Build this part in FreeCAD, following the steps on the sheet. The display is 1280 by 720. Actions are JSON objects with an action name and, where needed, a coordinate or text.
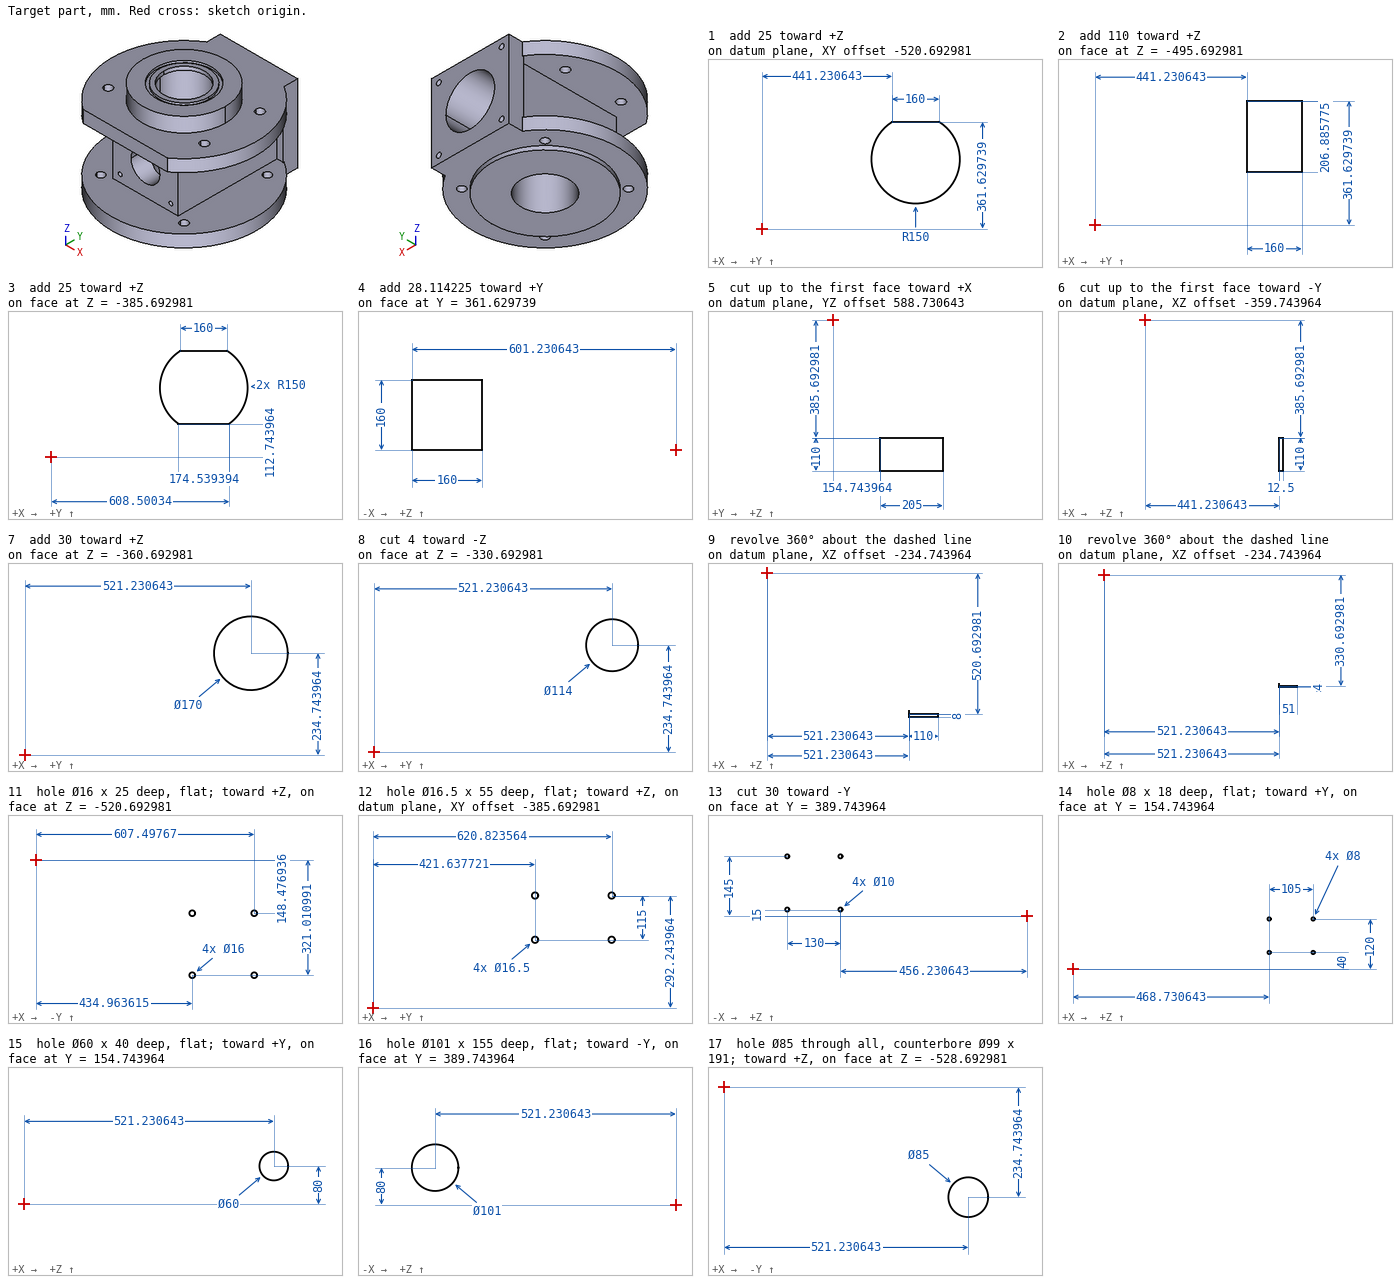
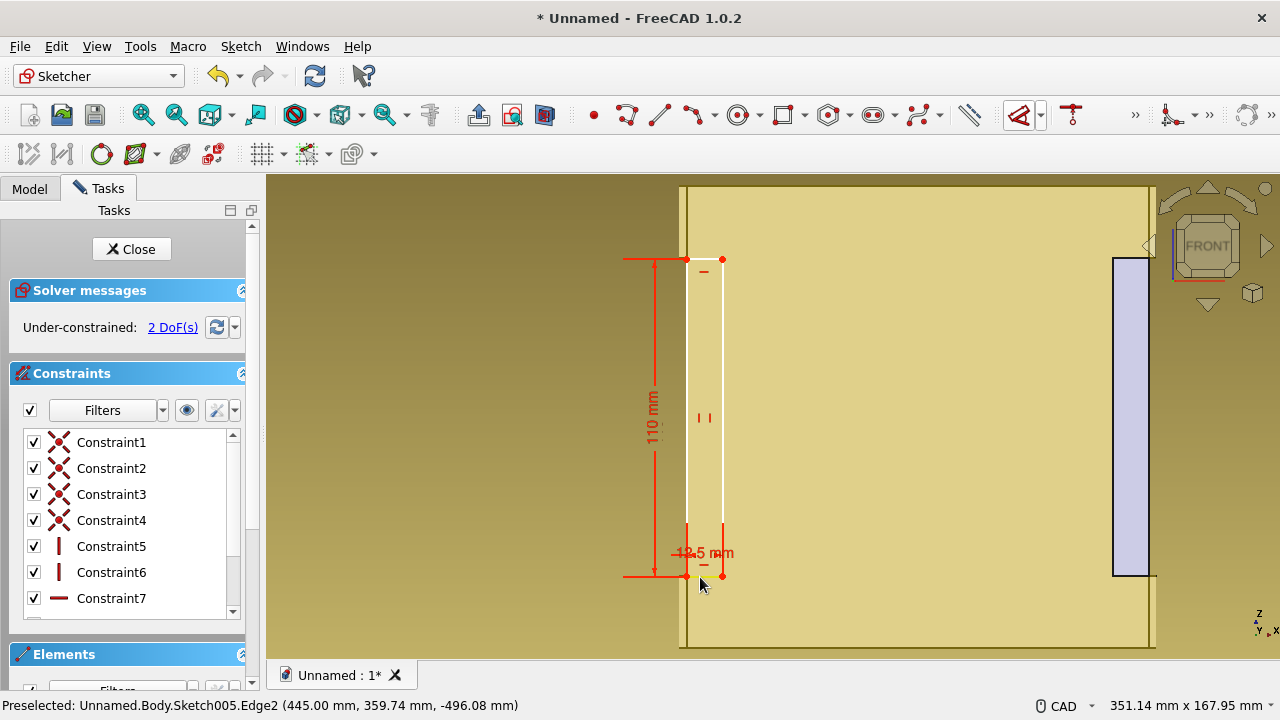
{"action": "left_click", "coordinate": [687, 259]}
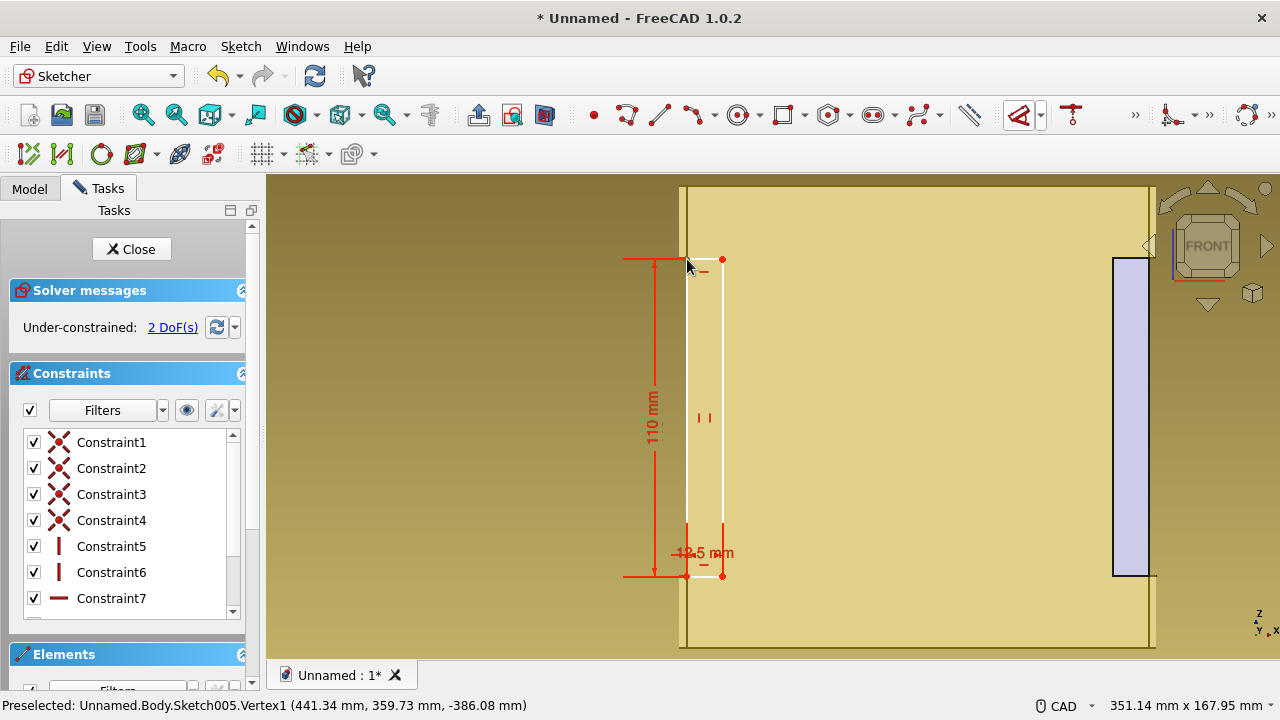
{"action": "left_click", "coordinate": [1040, 116]}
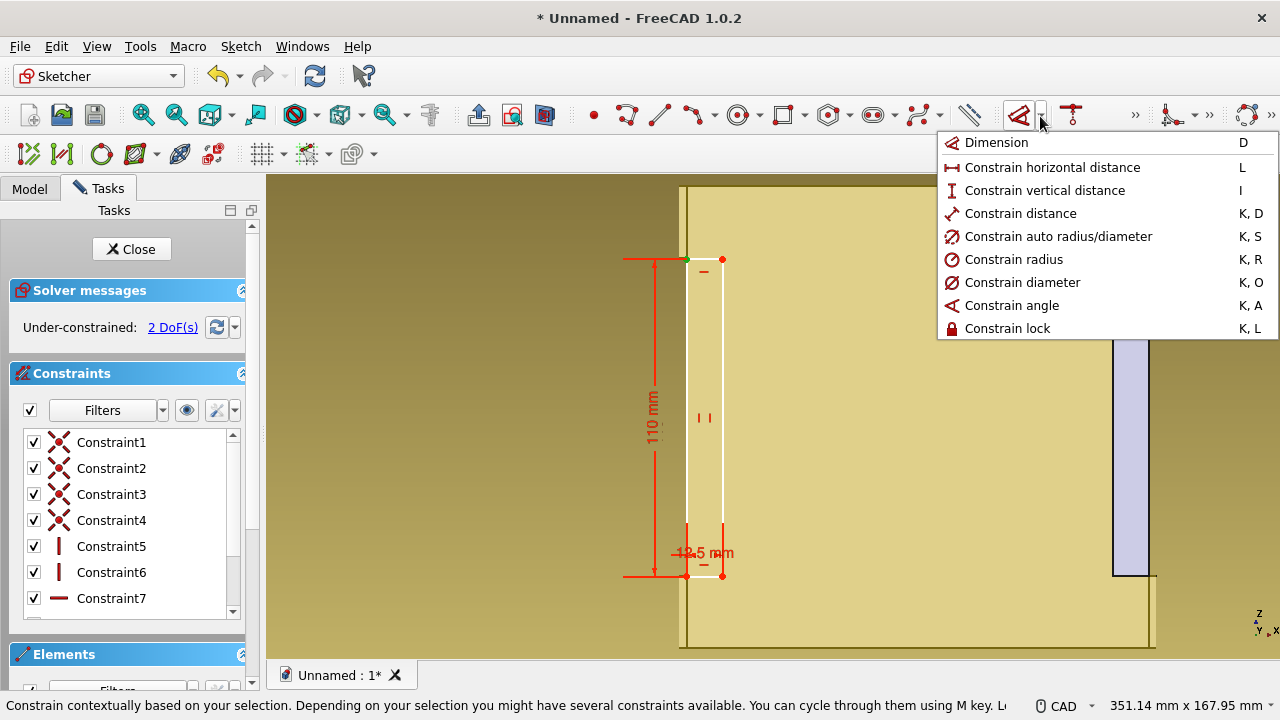
{"action": "left_click", "coordinate": [1108, 168]}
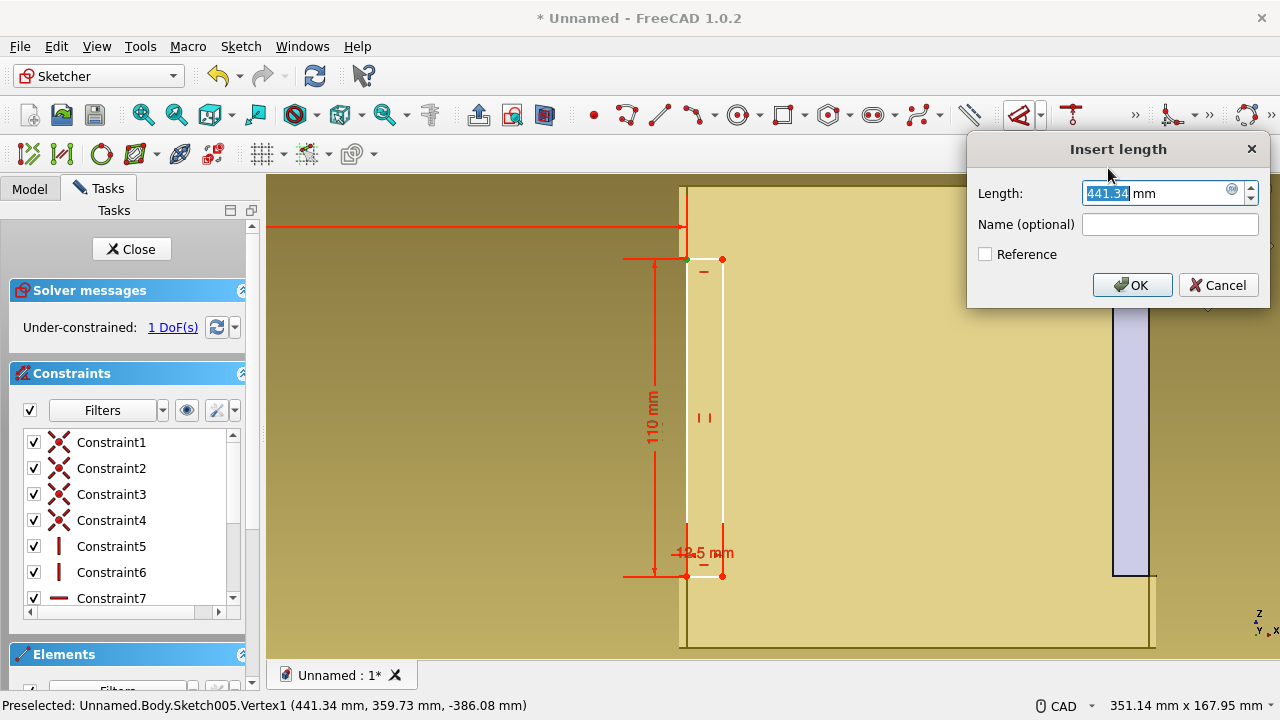
{"action": "type", "text": "441.230643"}
{"action": "key", "text": "Return"}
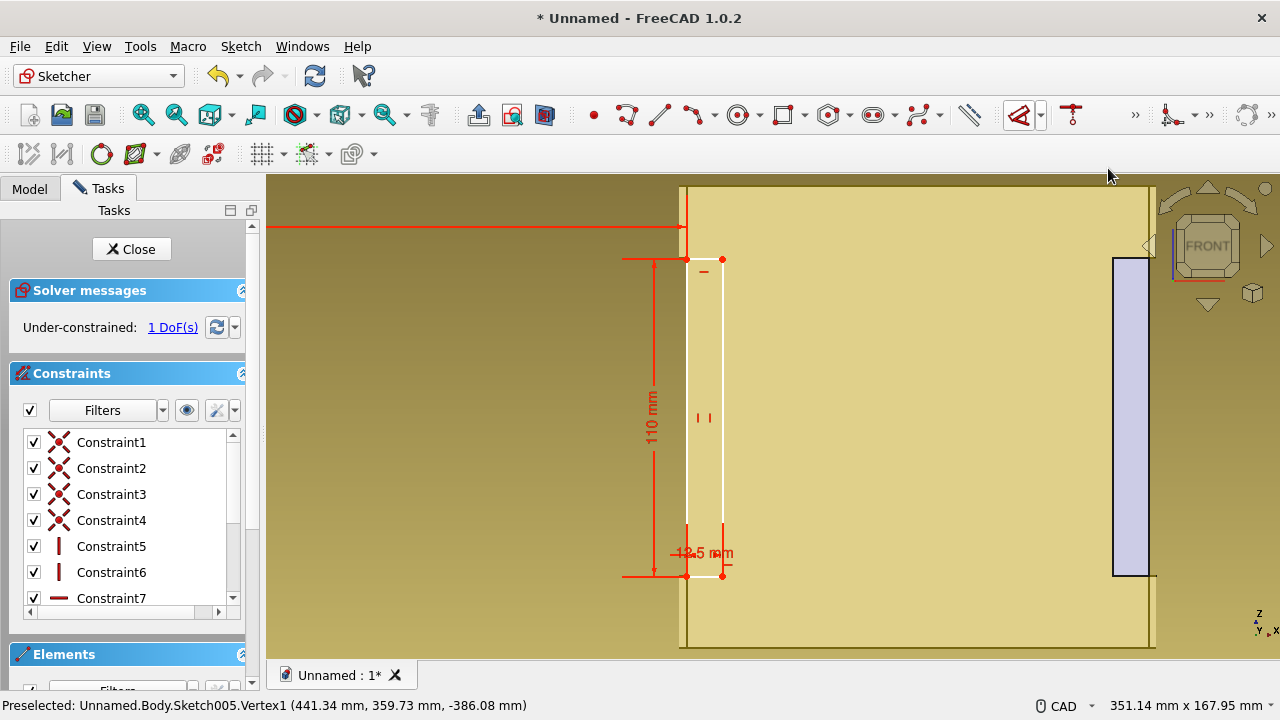
{"action": "left_click", "coordinate": [687, 259]}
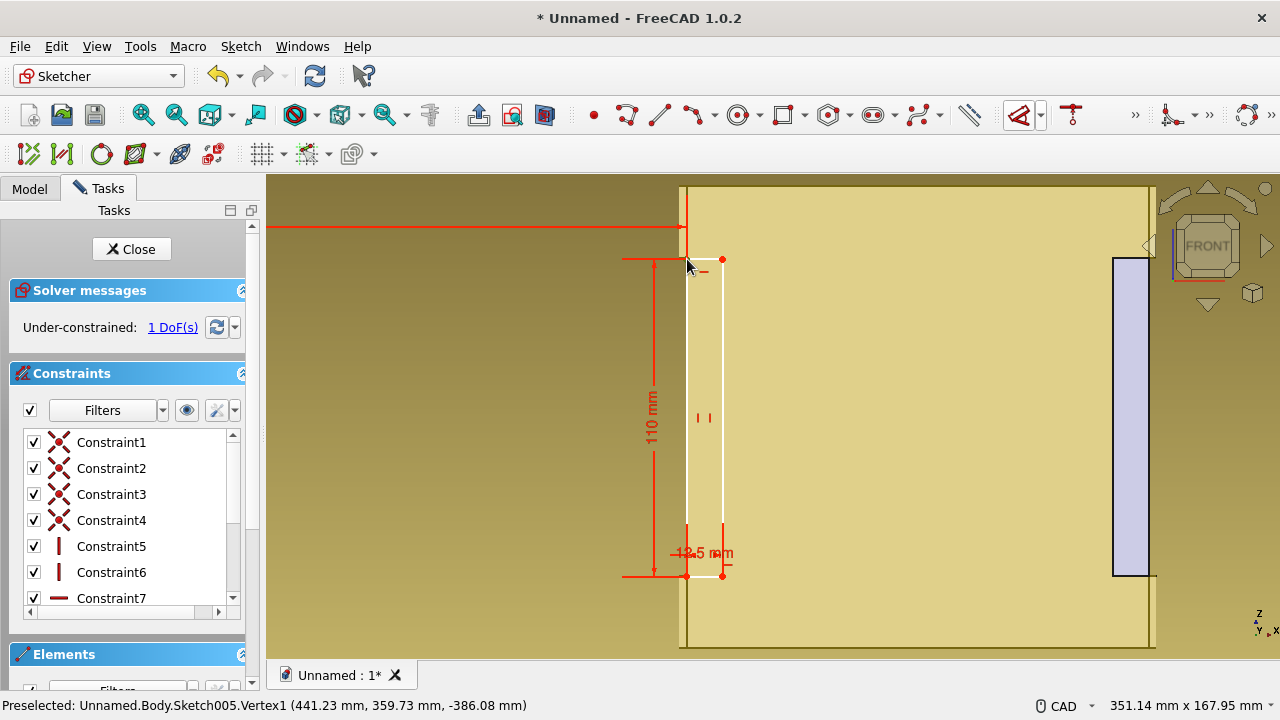
{"action": "left_click", "coordinate": [1040, 116]}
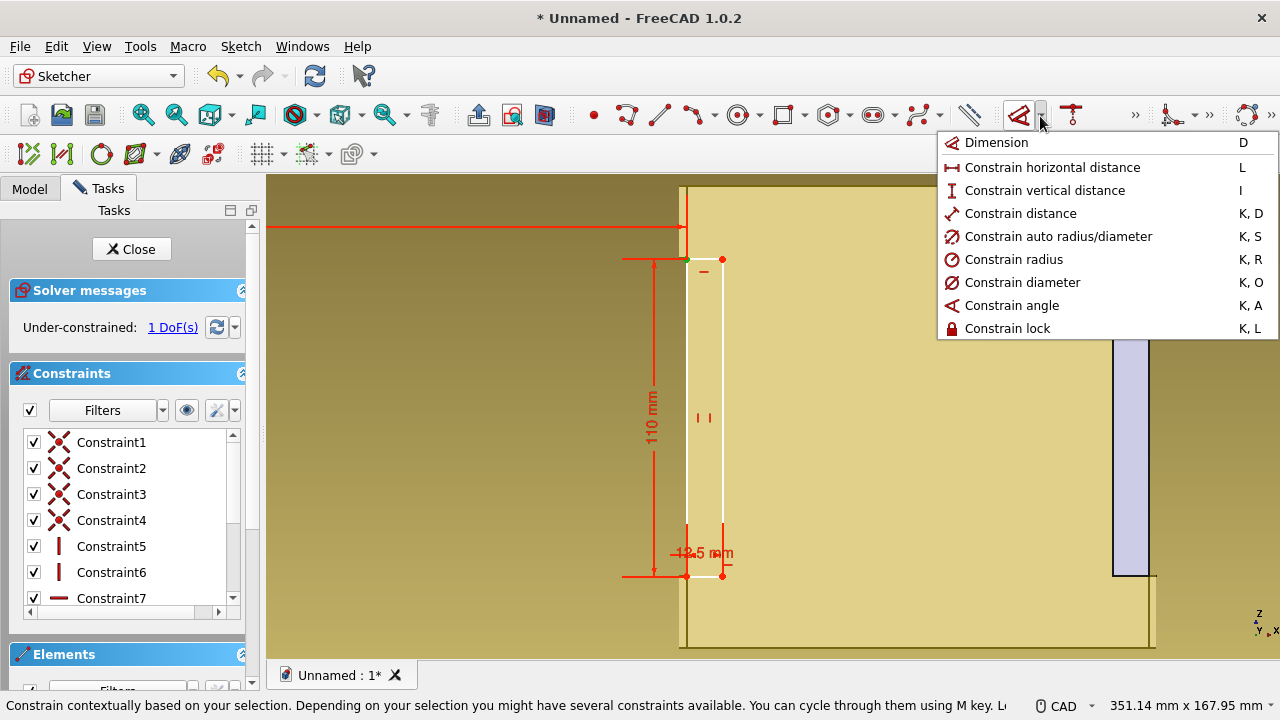
{"action": "left_click", "coordinate": [1108, 190]}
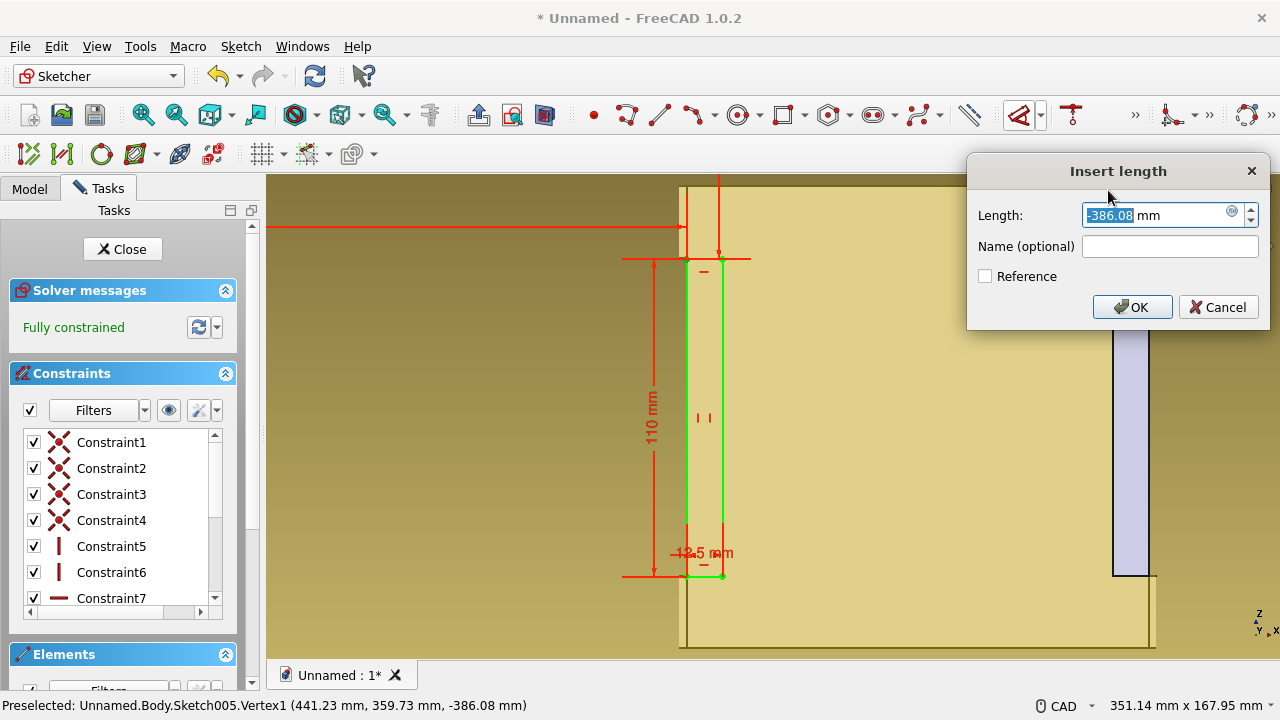
{"action": "type", "text": "-385.692981"}
{"action": "key", "text": "Return"}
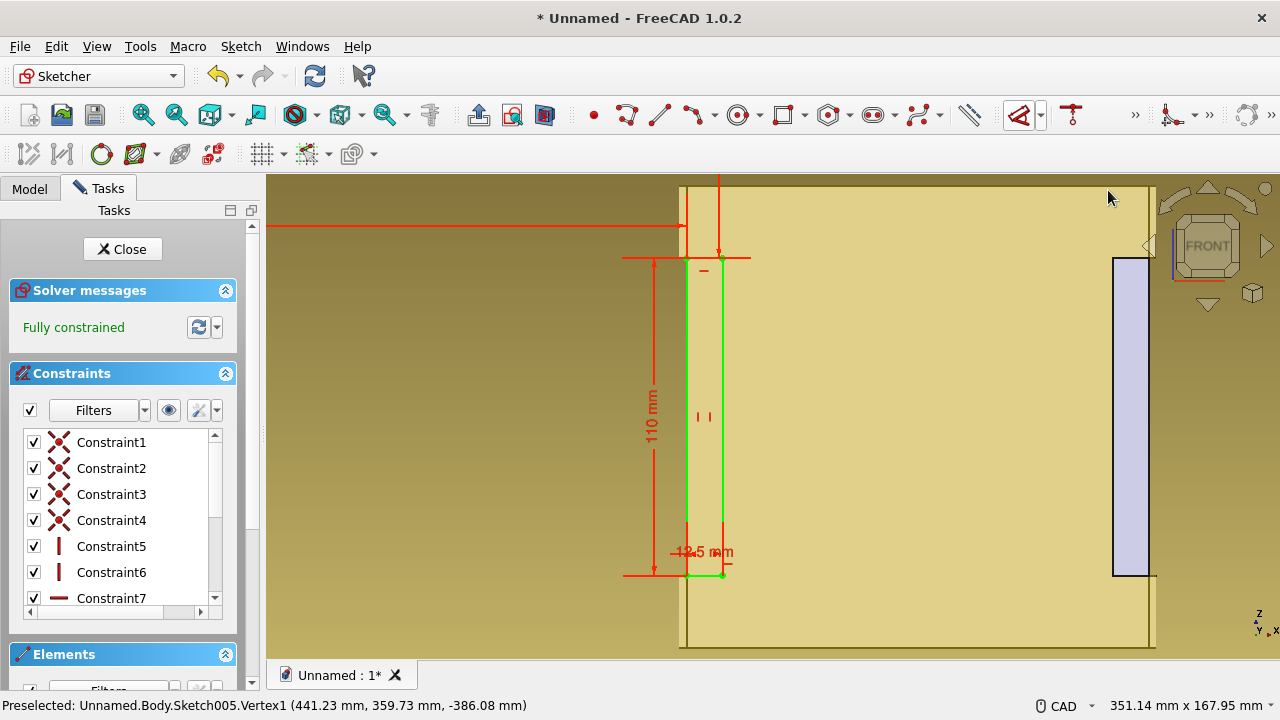
{"action": "left_click", "coordinate": [123, 249]}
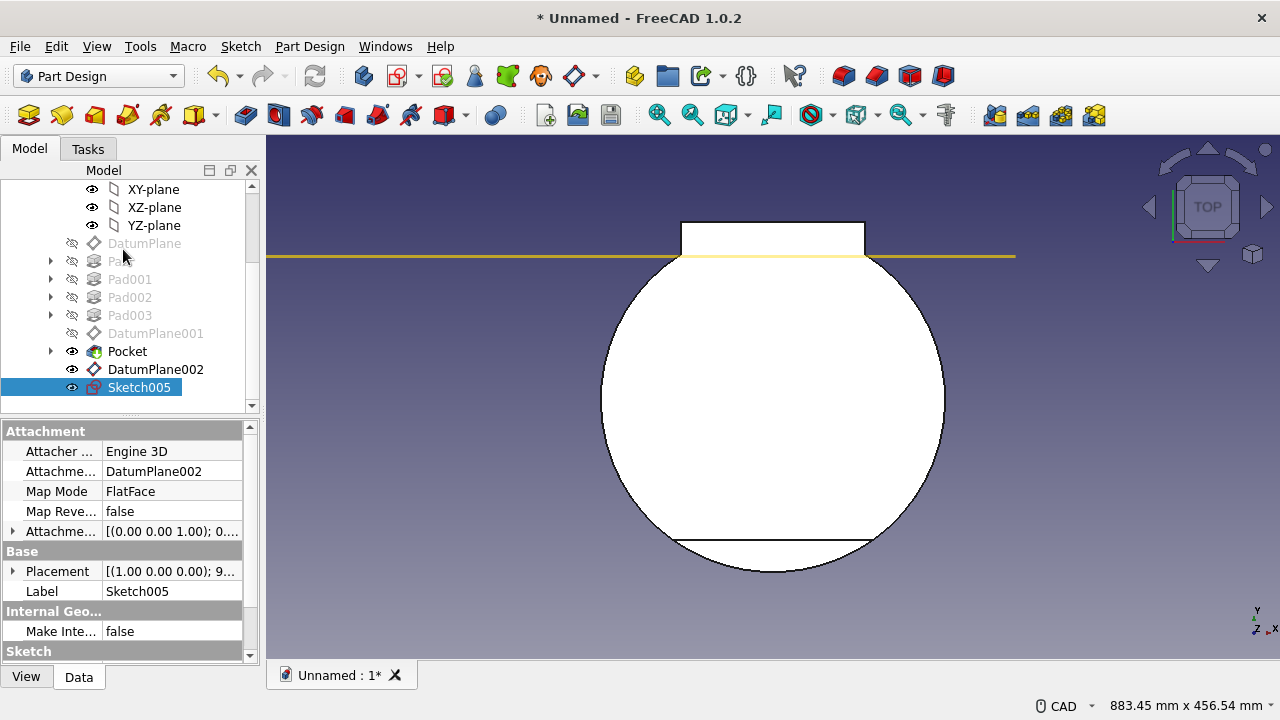
{"action": "left_click", "coordinate": [246, 116]}